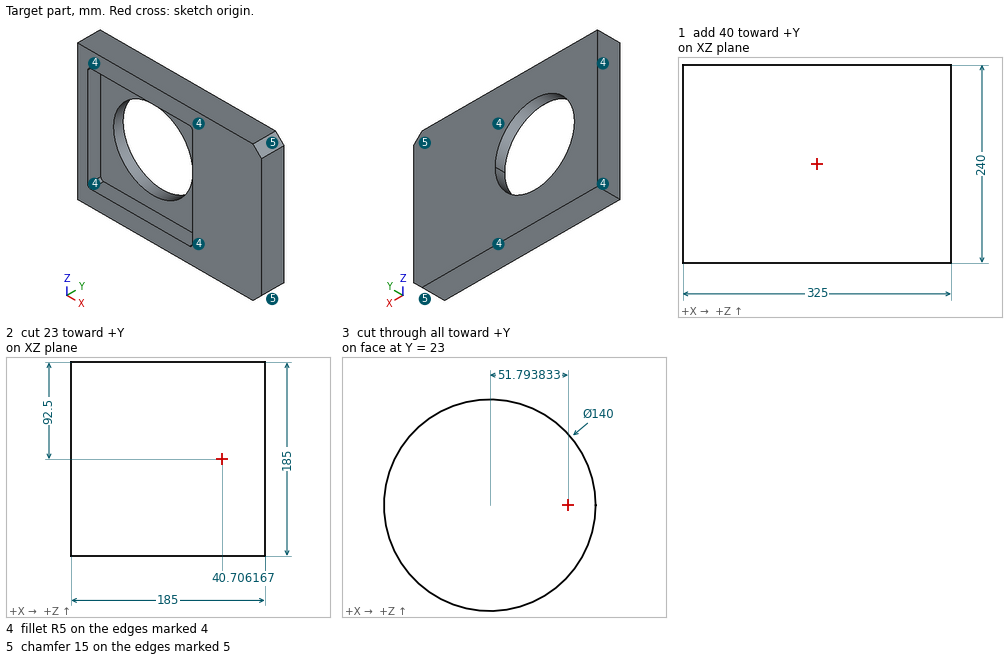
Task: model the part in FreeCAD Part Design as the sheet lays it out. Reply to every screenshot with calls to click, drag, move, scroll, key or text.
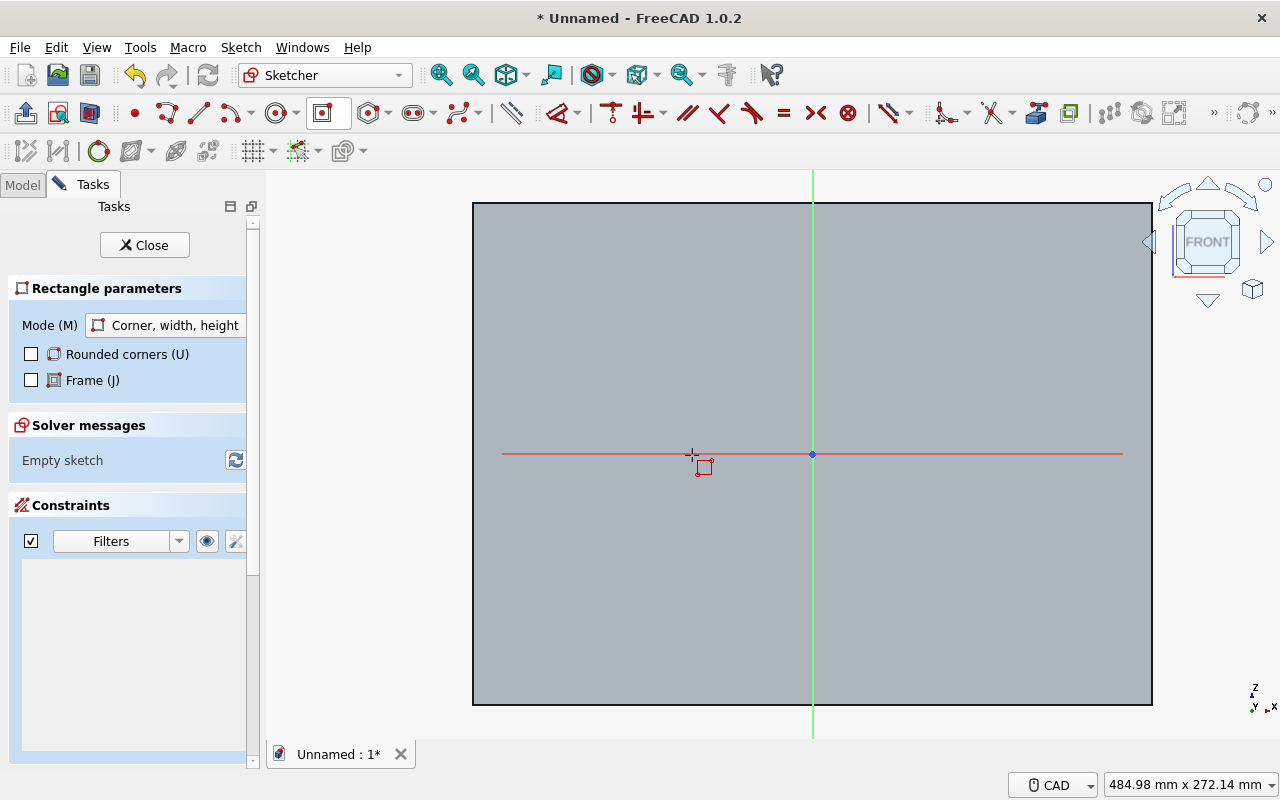
click(511, 261)
move(898, 647)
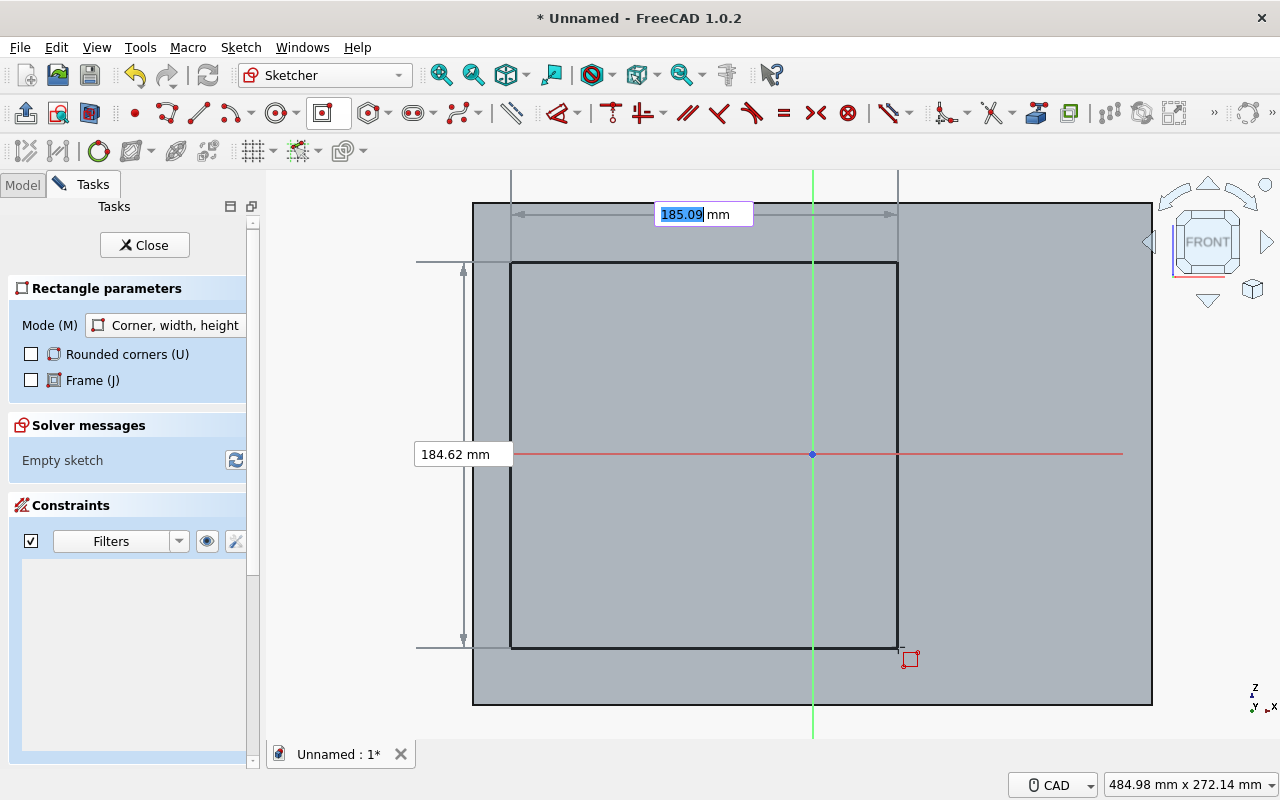
text(185)
key(Tab)
text(185)
key(Return)
key(Escape)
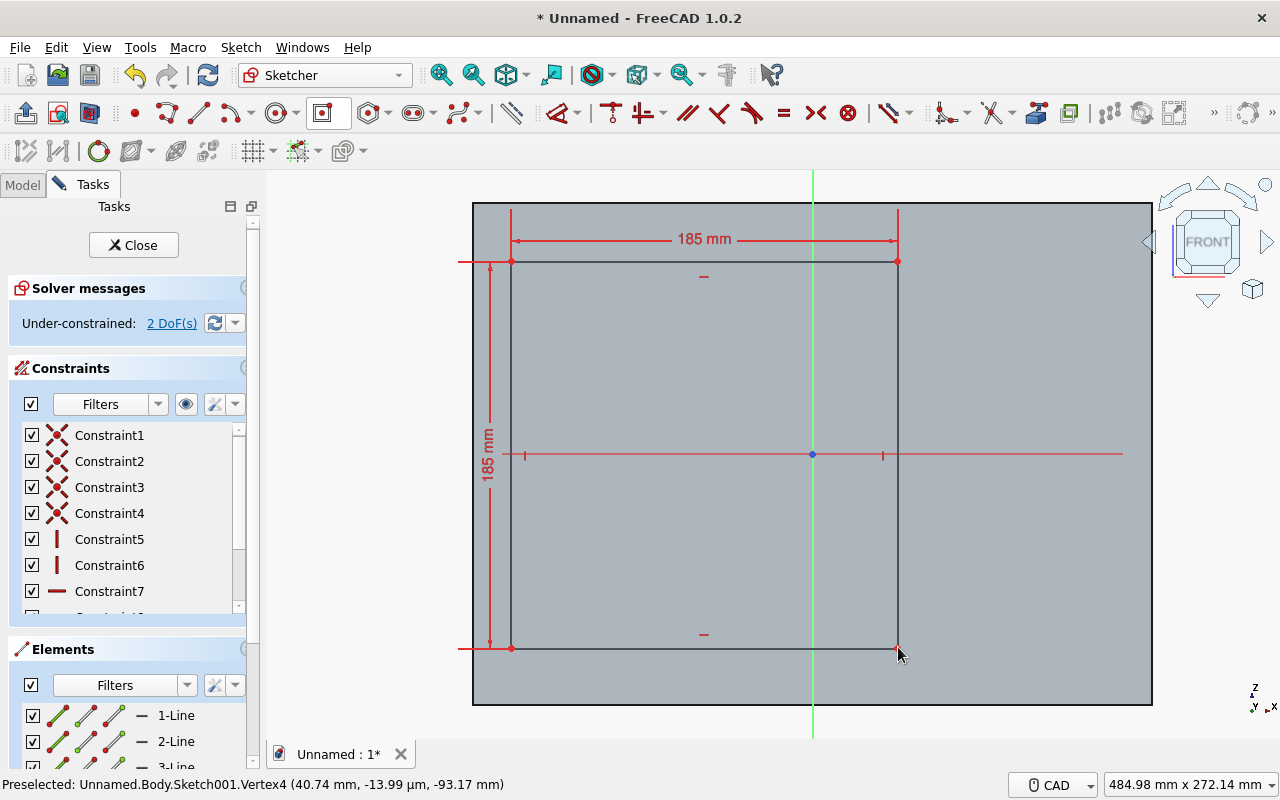
click(558, 114)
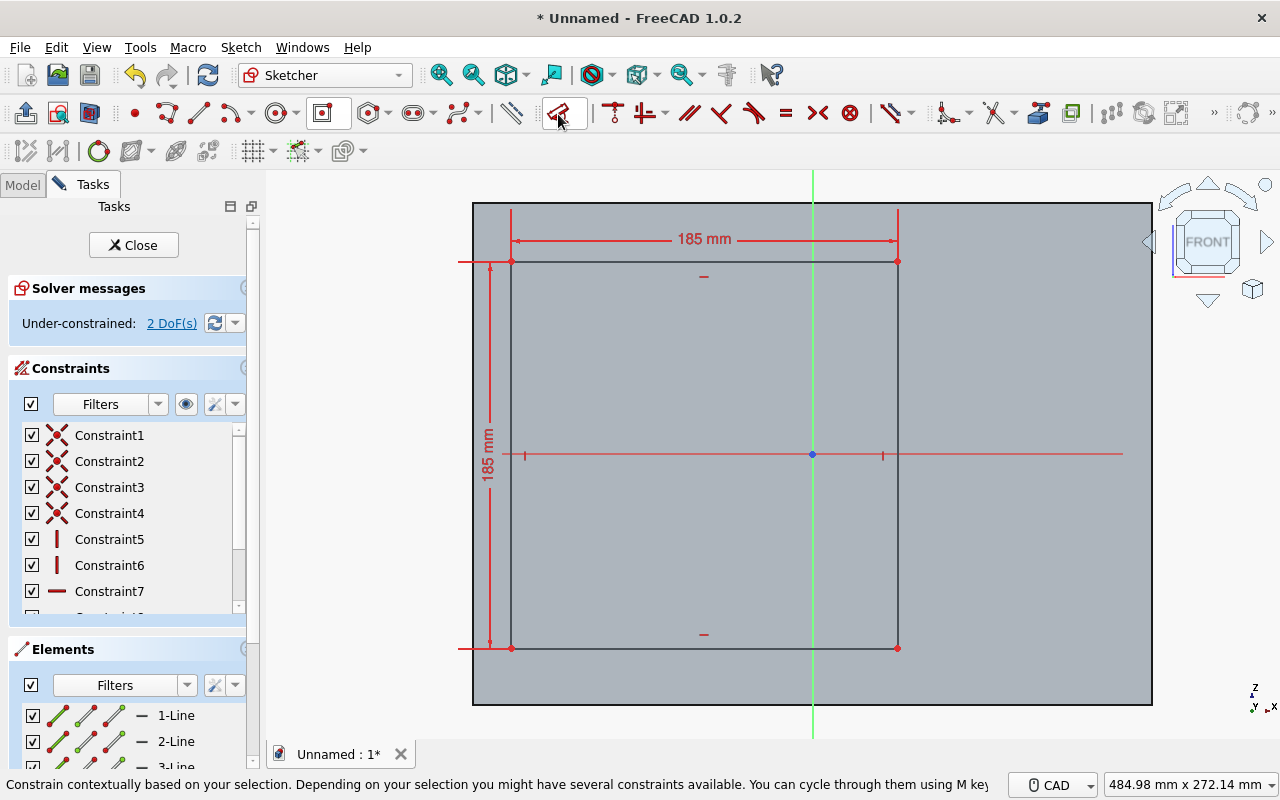
click(511, 262)
click(477, 358)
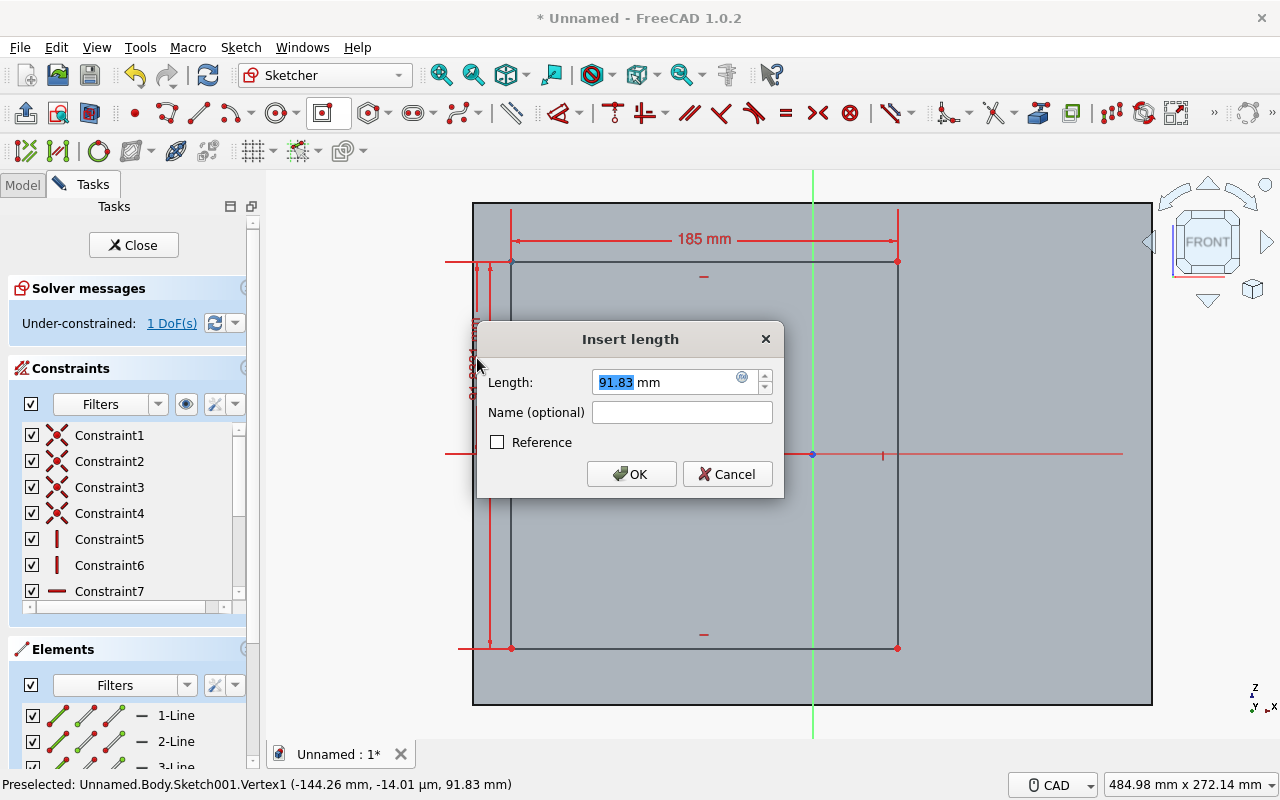
text(92.5)
key(Return)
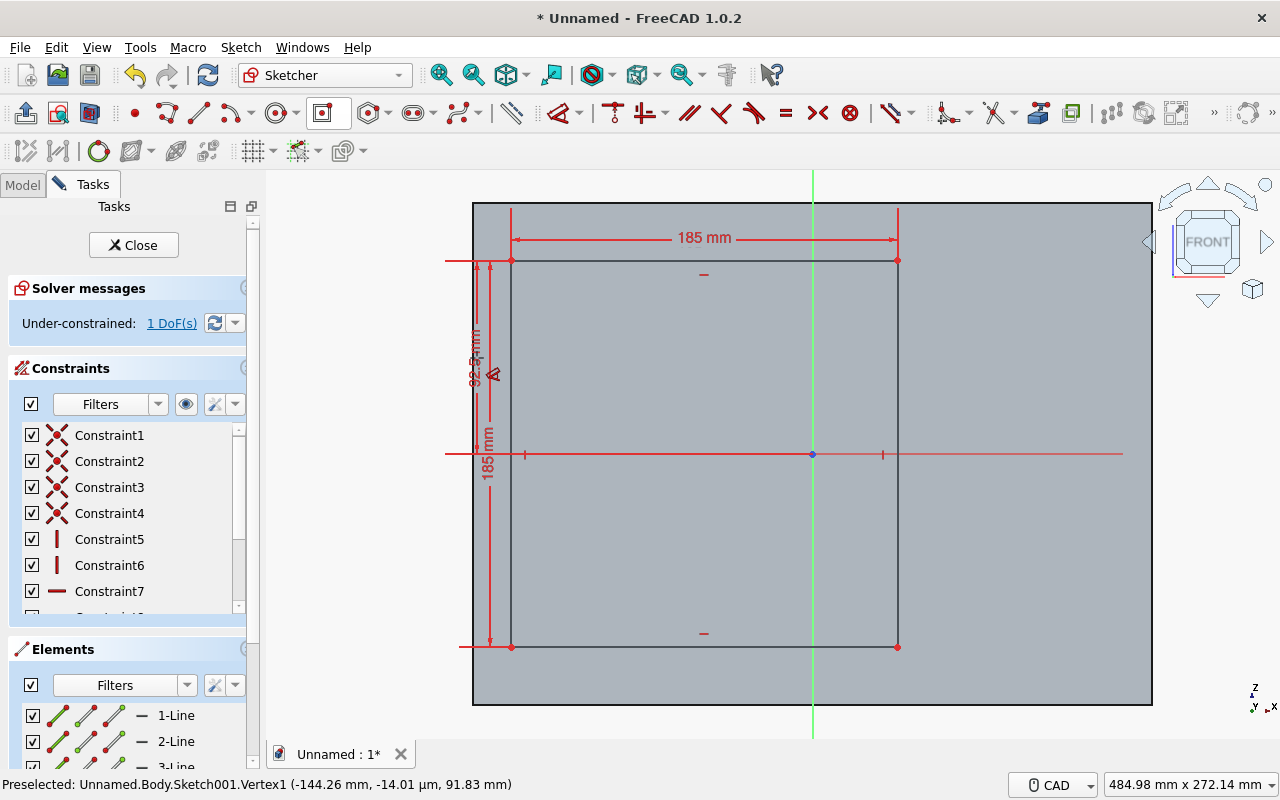
click(898, 647)
click(855, 681)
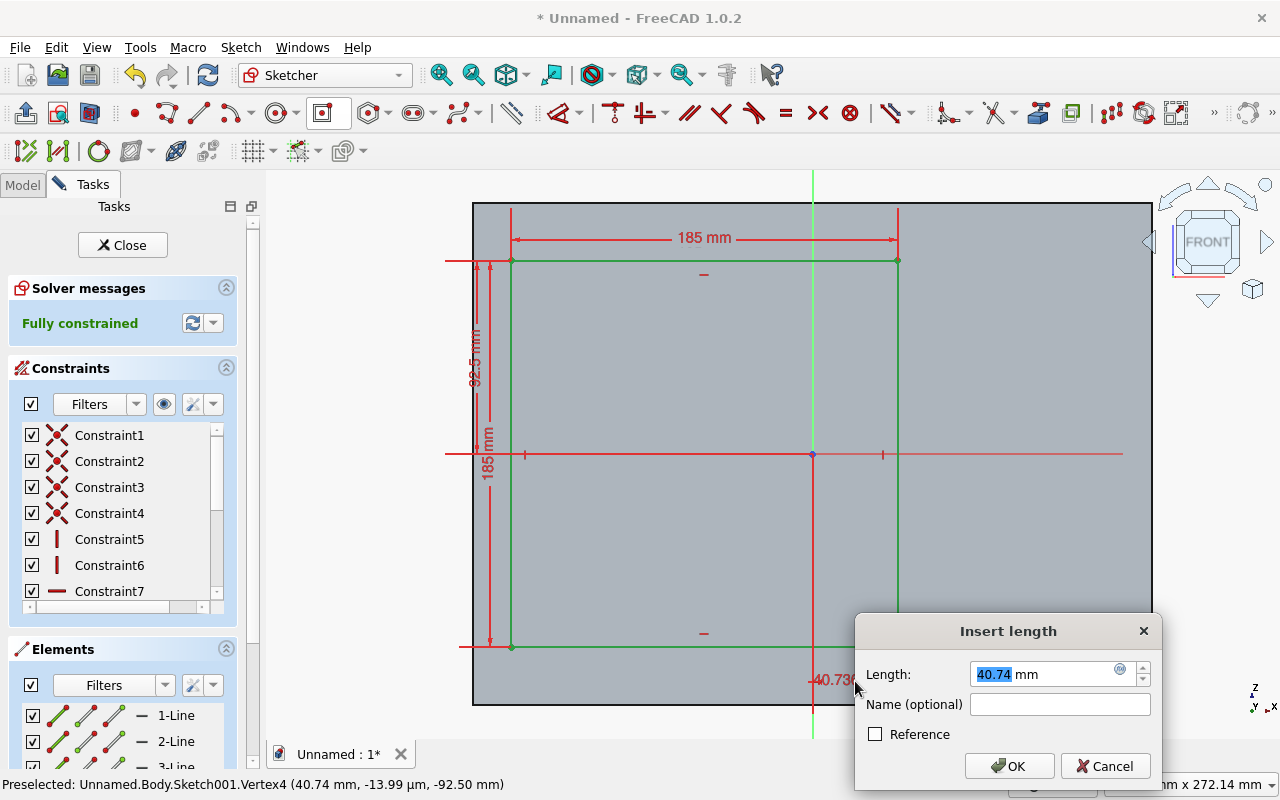
text(40.706167)
key(Return)
key(Escape)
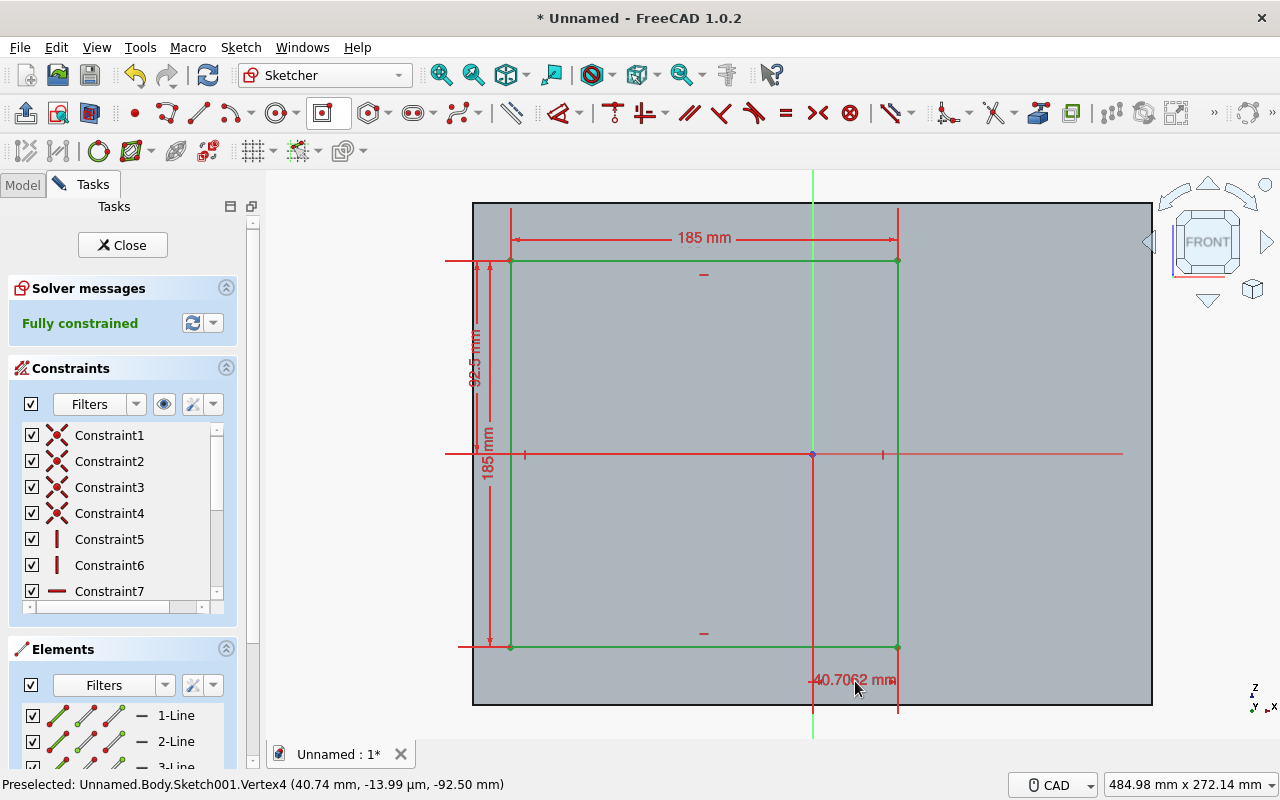
click(123, 245)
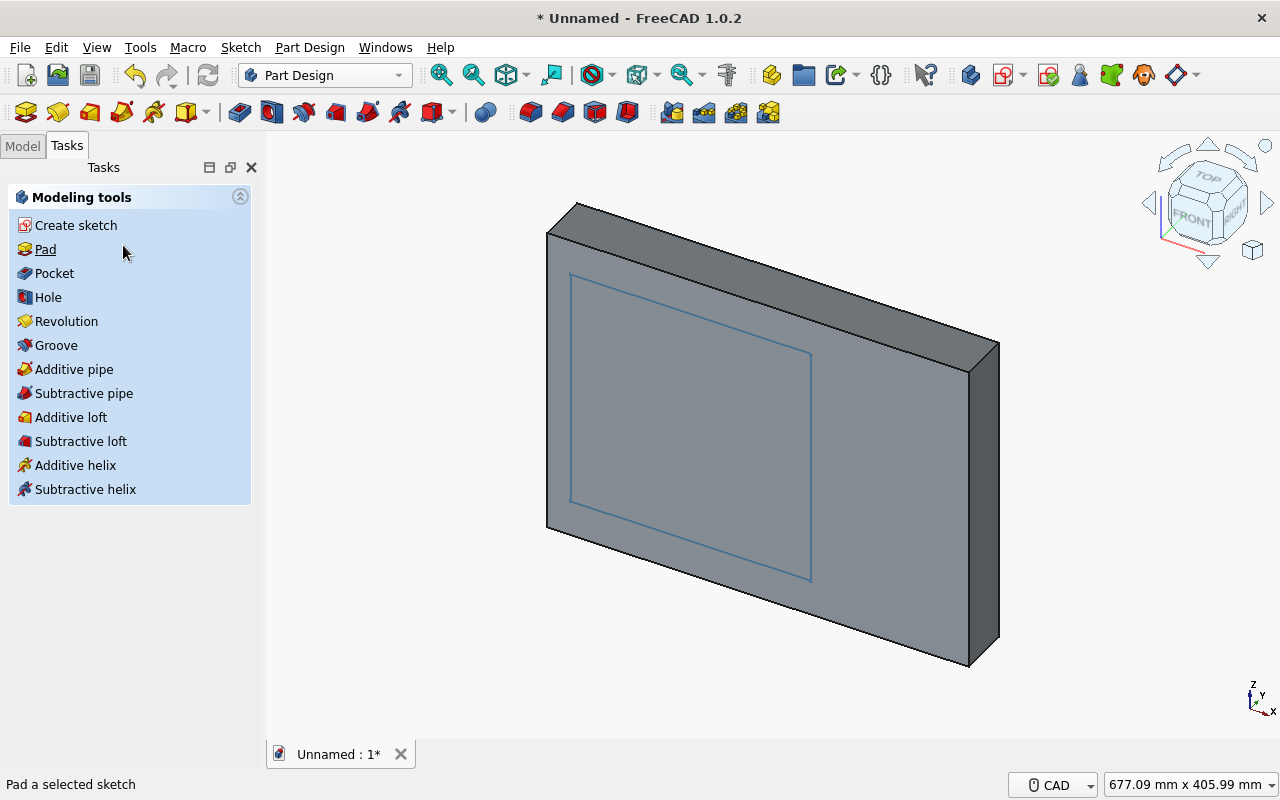
click(240, 112)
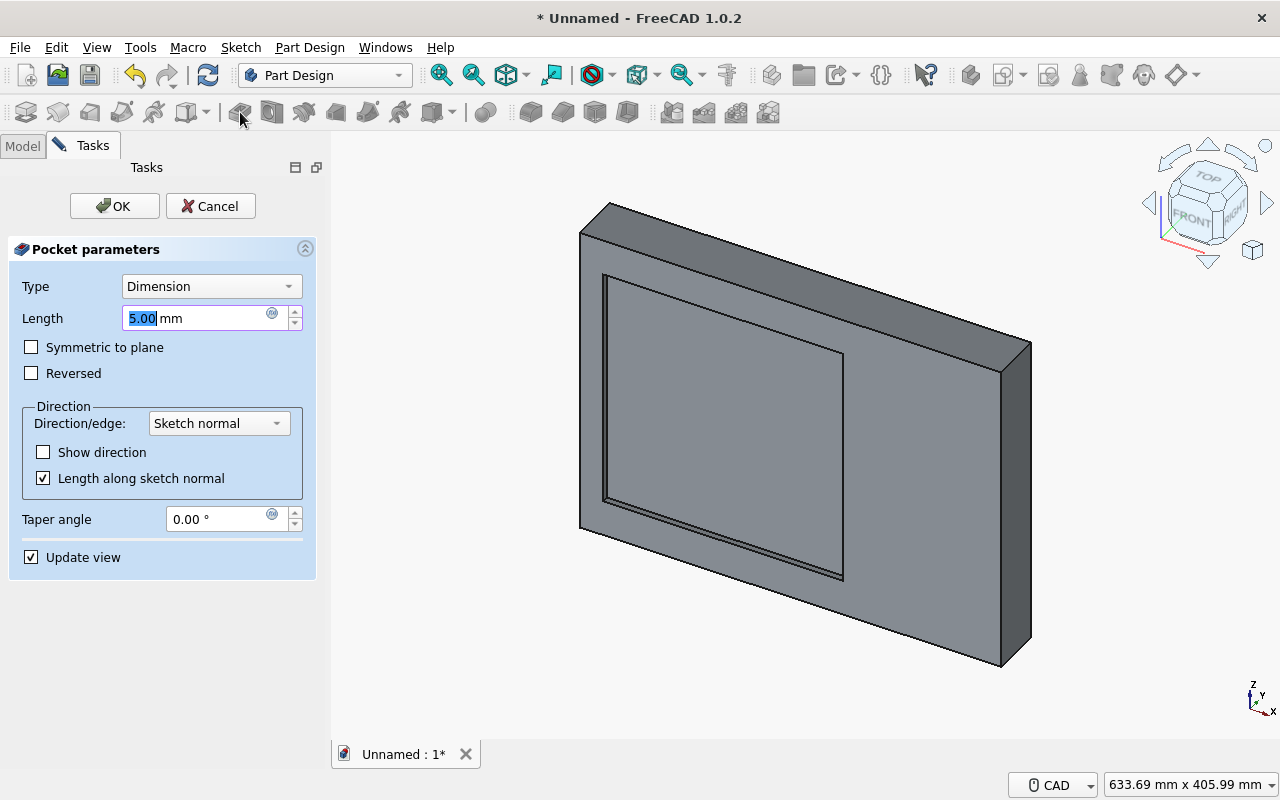
text(23)
key(Tab)